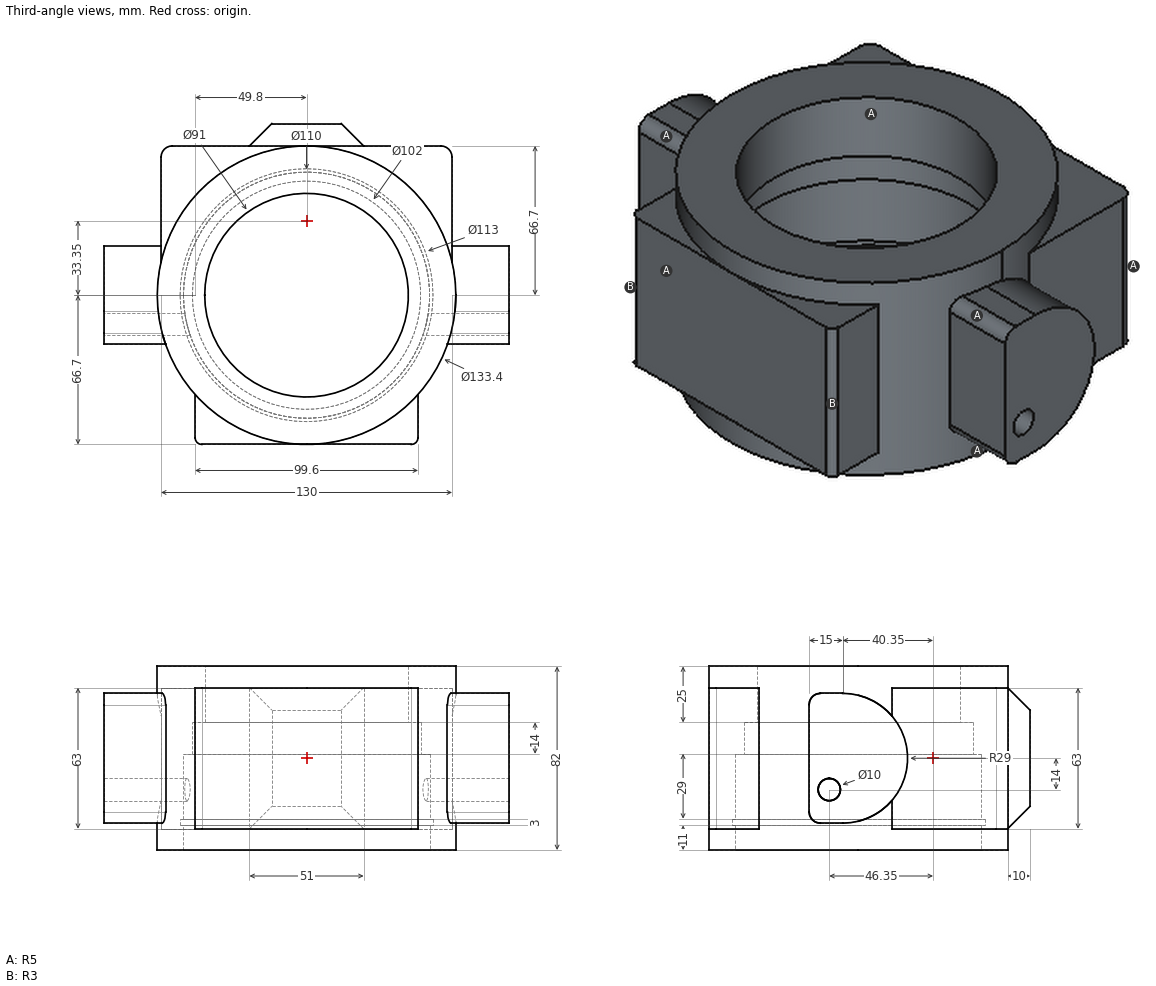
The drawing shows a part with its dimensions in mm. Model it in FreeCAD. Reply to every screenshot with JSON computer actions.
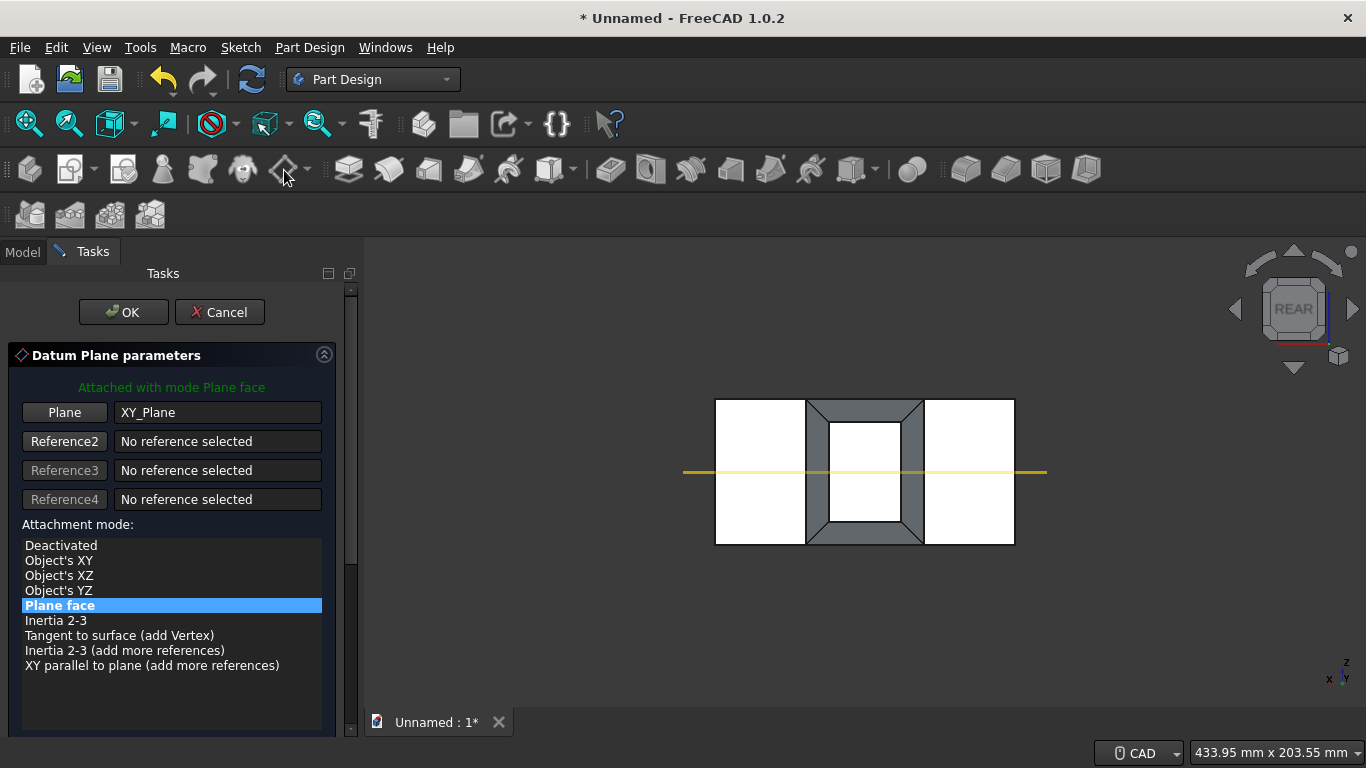
{"action": "scroll", "coordinate": [351, 510], "scroll_direction": "down", "scroll_amount": 3}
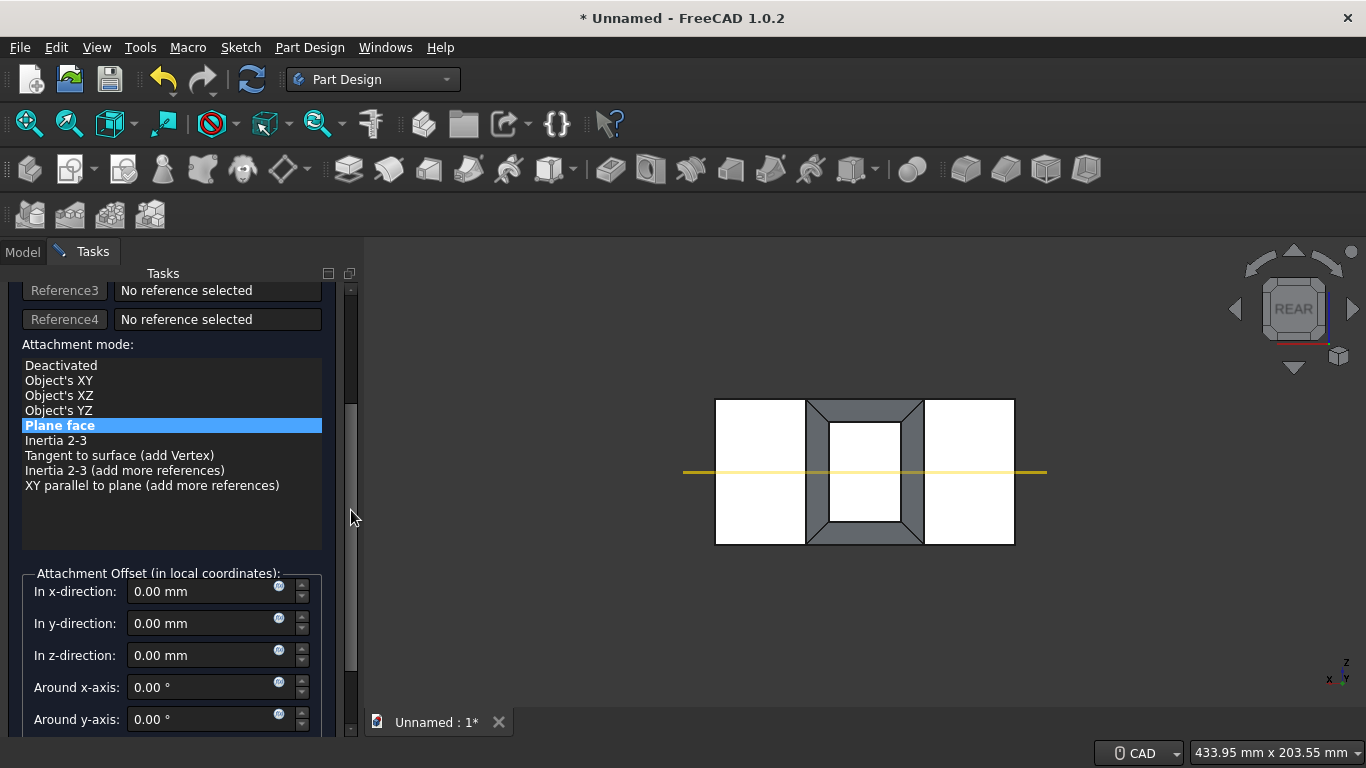
{"action": "triple_click", "coordinate": [210, 655]}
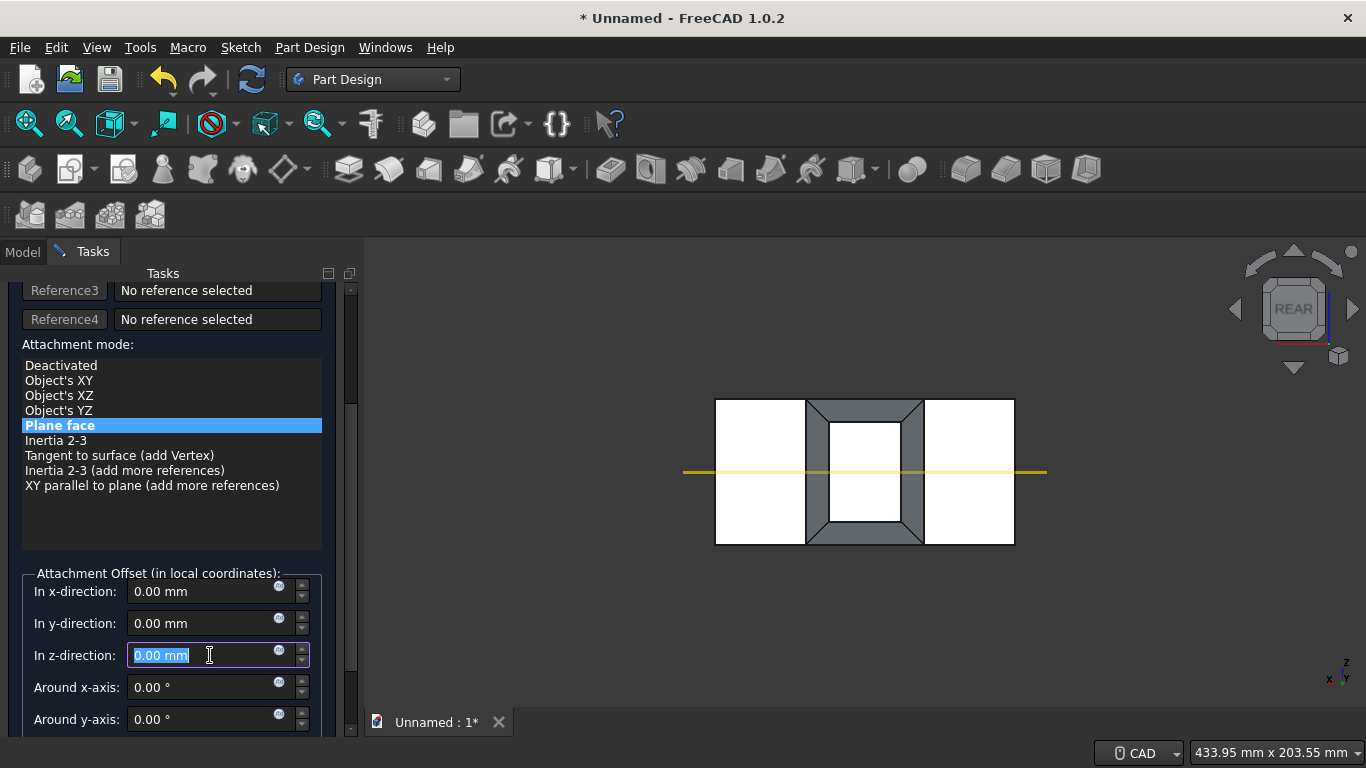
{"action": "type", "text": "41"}
{"action": "key", "text": "Tab"}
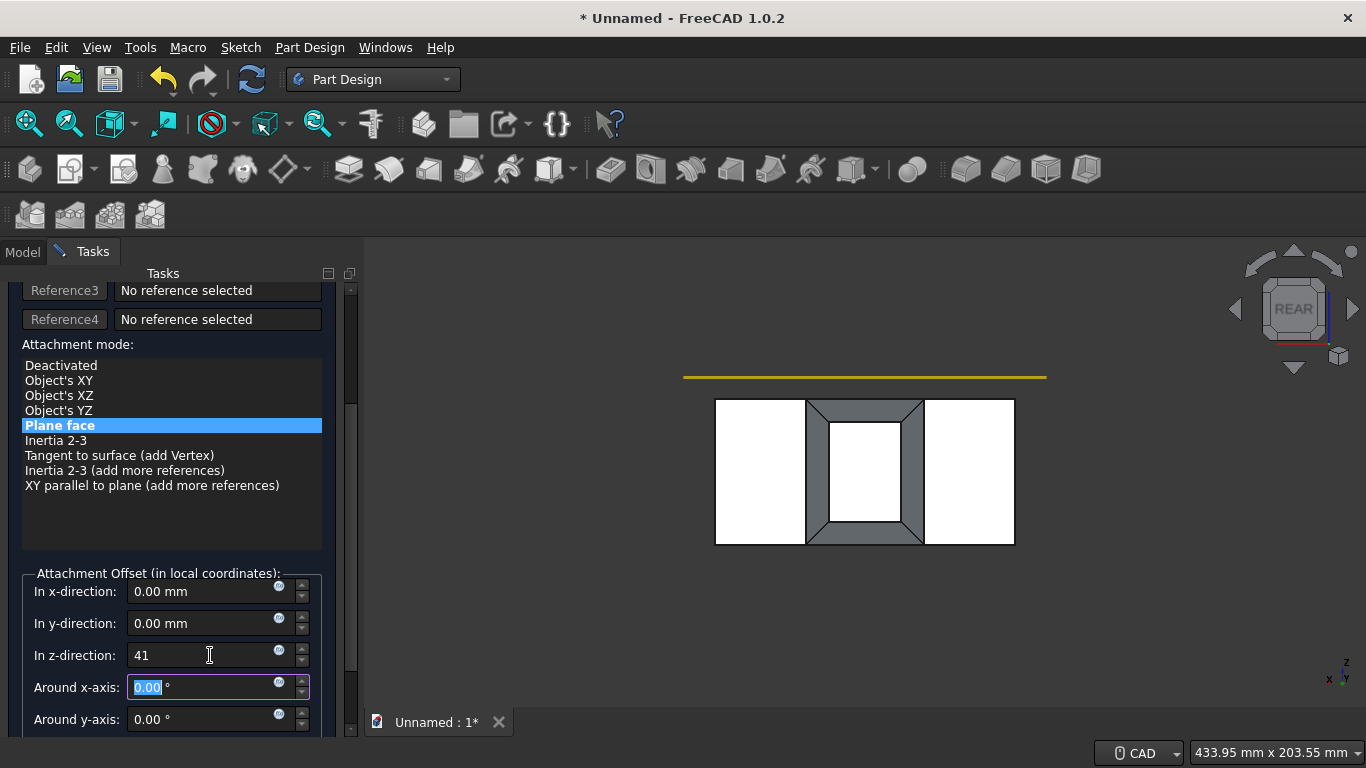
{"action": "scroll", "coordinate": [351, 510], "scroll_direction": "up", "scroll_amount": 4}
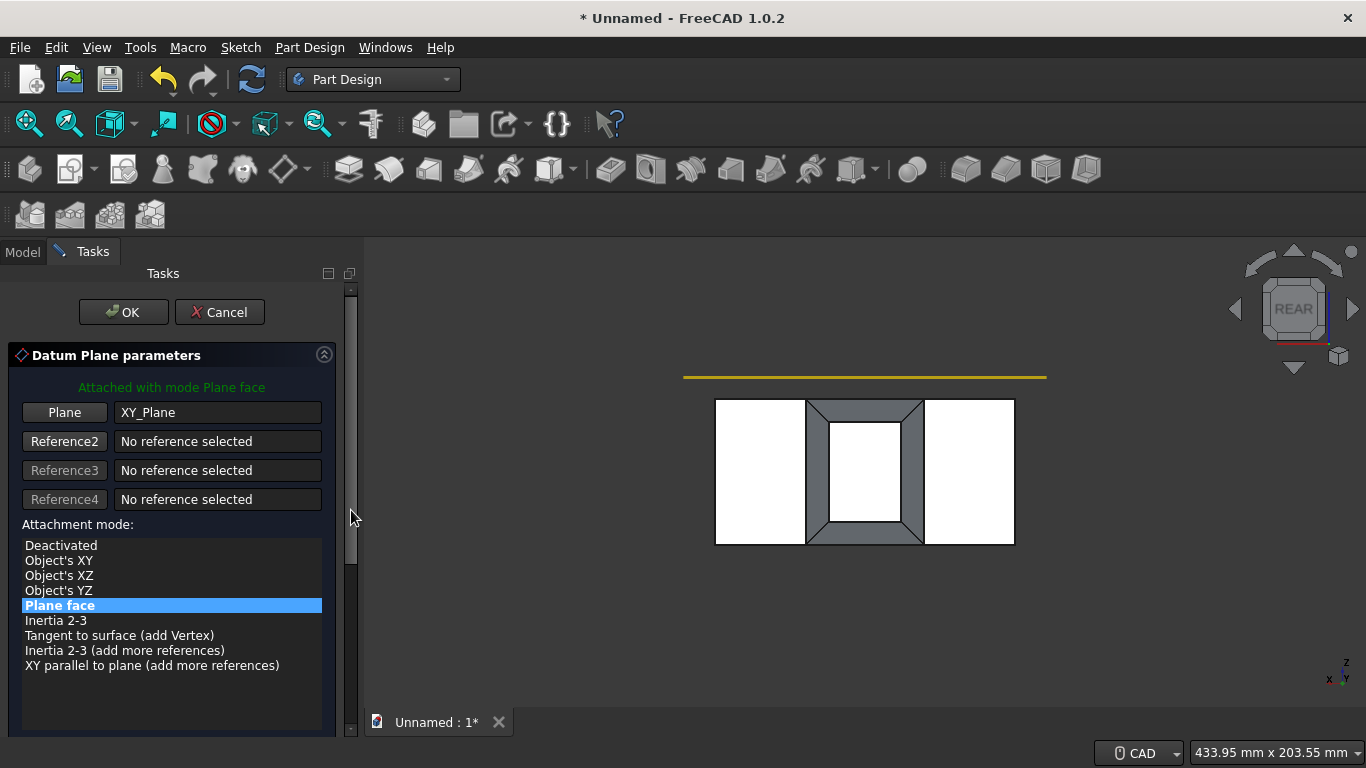
{"action": "left_click", "coordinate": [124, 312]}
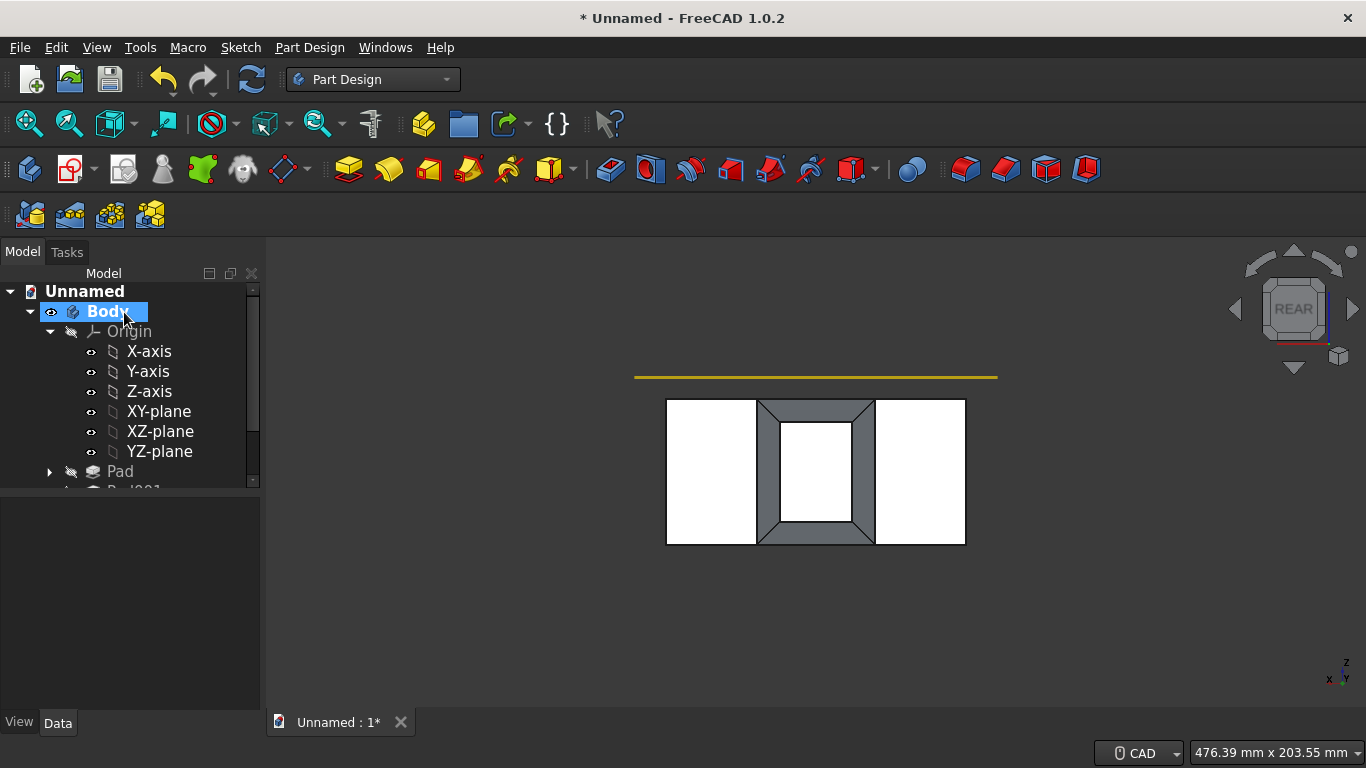
{"action": "scroll", "coordinate": [100, 387], "scroll_direction": "down", "scroll_amount": 3}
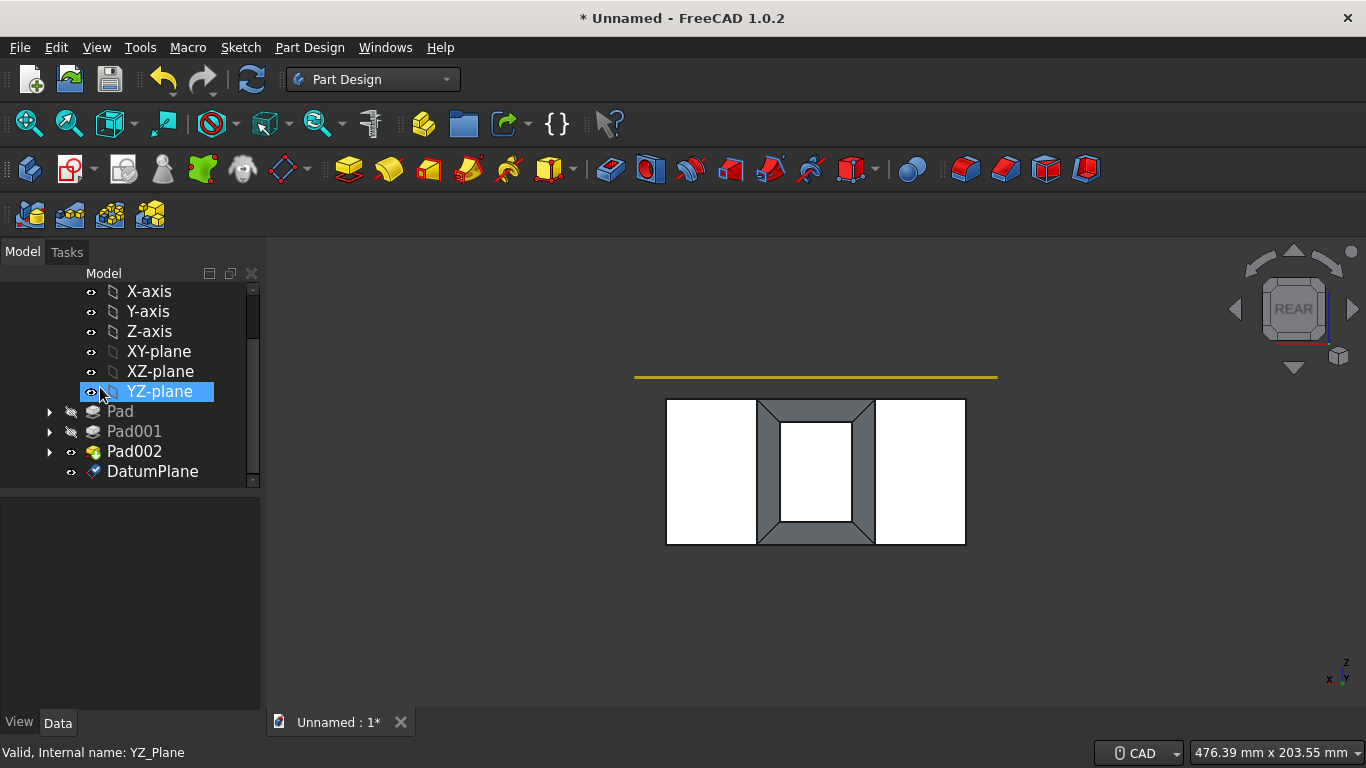
{"action": "left_click", "coordinate": [116, 472]}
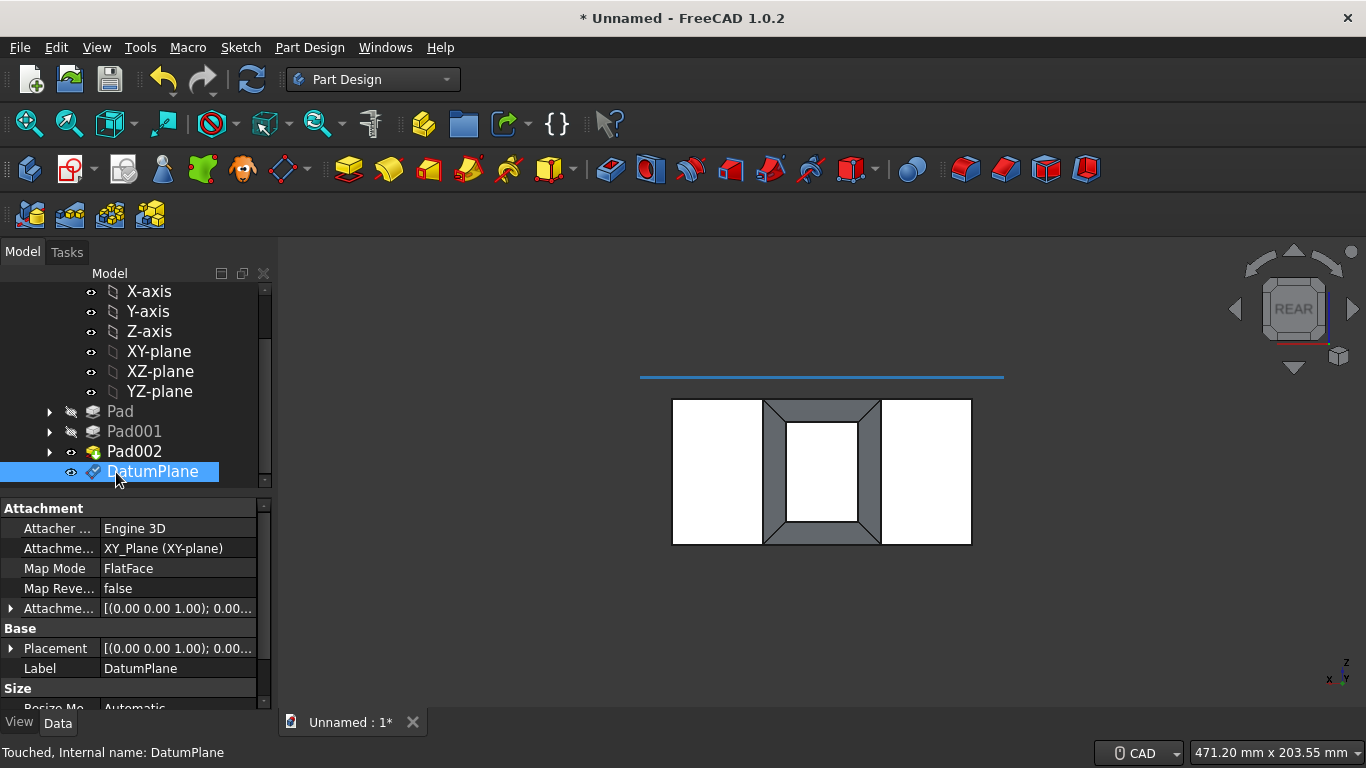
{"action": "left_click", "coordinate": [70, 170]}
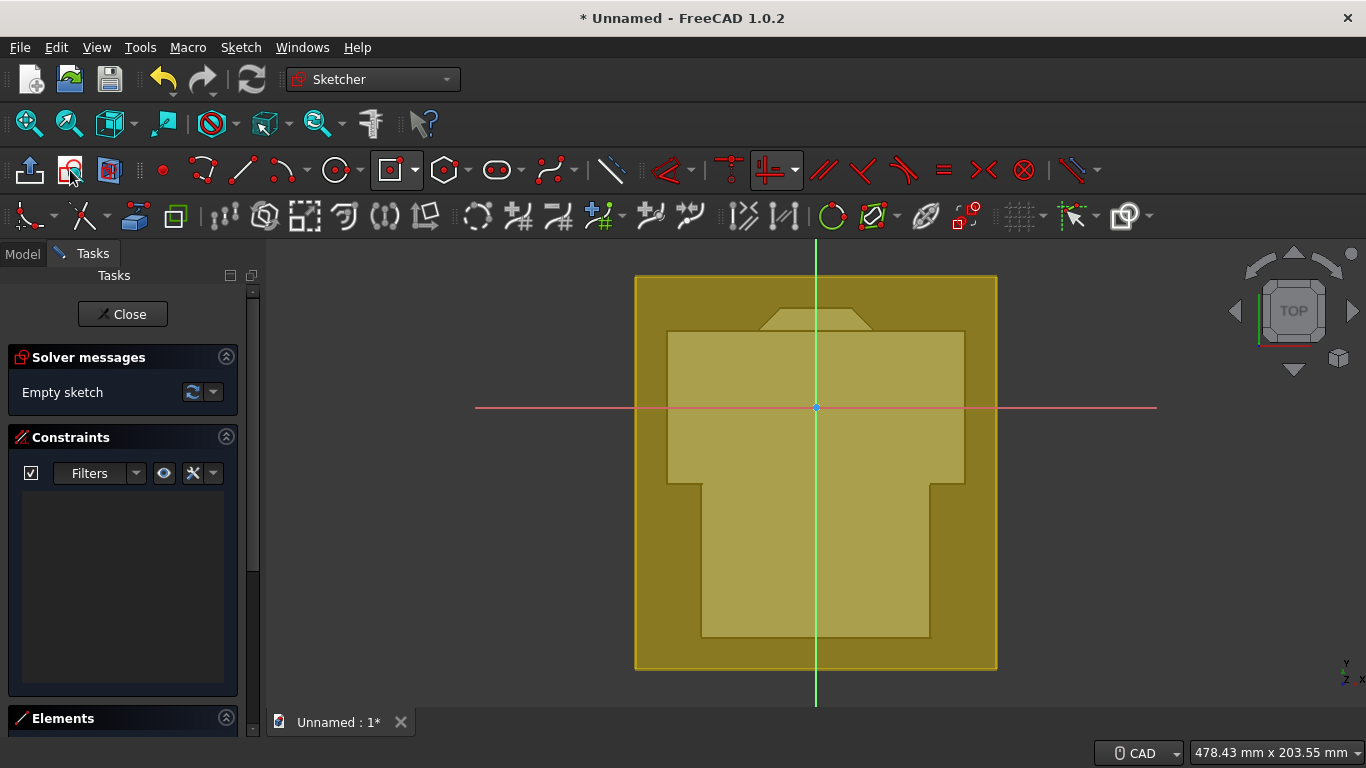
{"action": "left_click", "coordinate": [336, 170]}